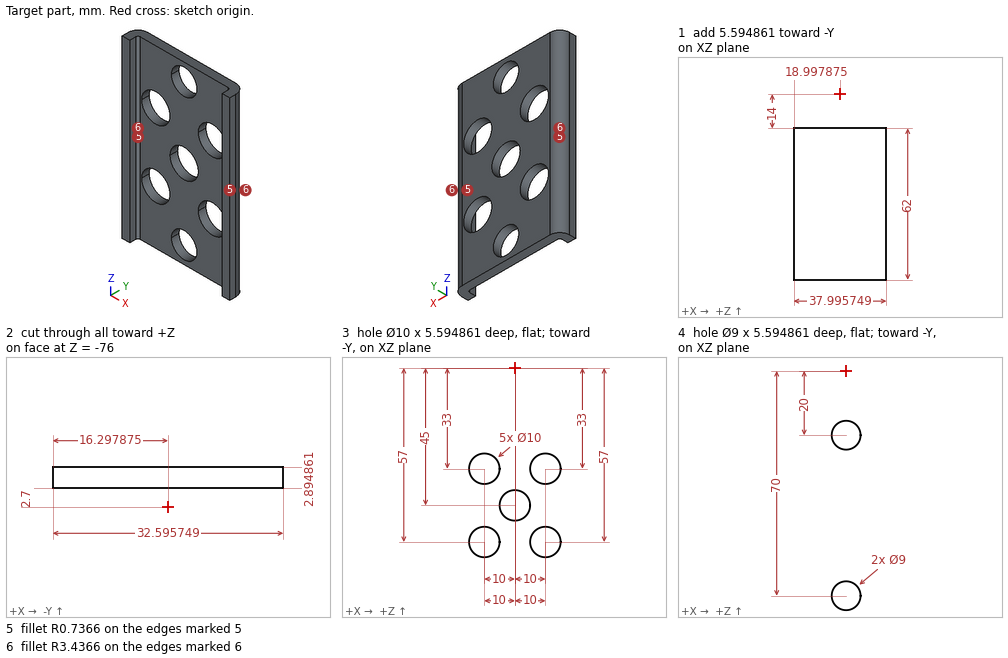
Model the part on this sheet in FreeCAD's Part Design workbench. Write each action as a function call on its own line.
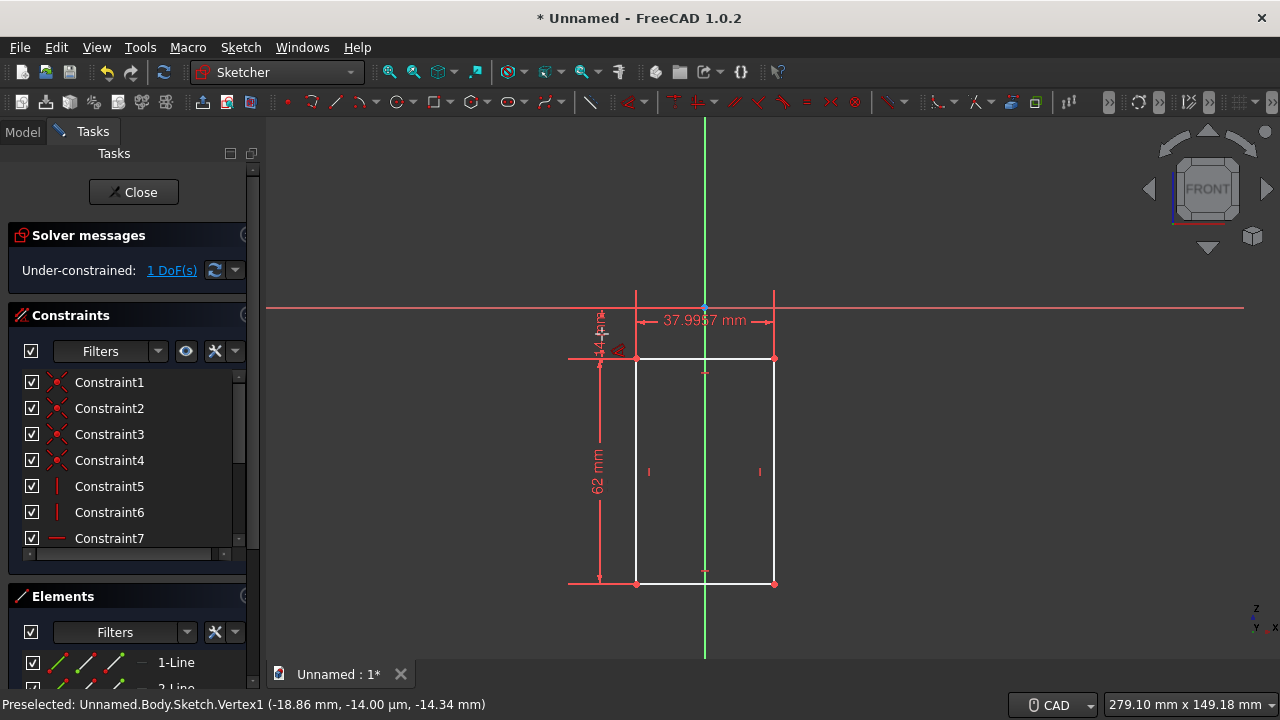
click(636, 359)
click(670, 274)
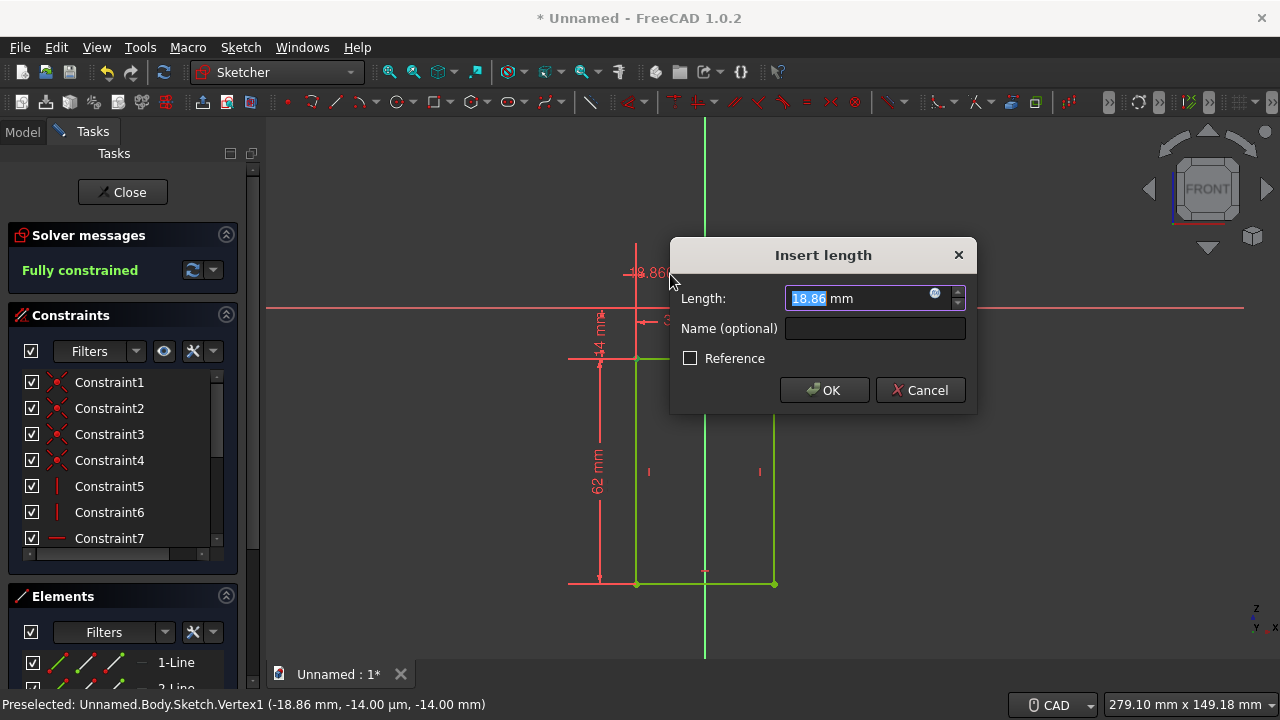
text(18.997875)
key(Return)
key(Escape)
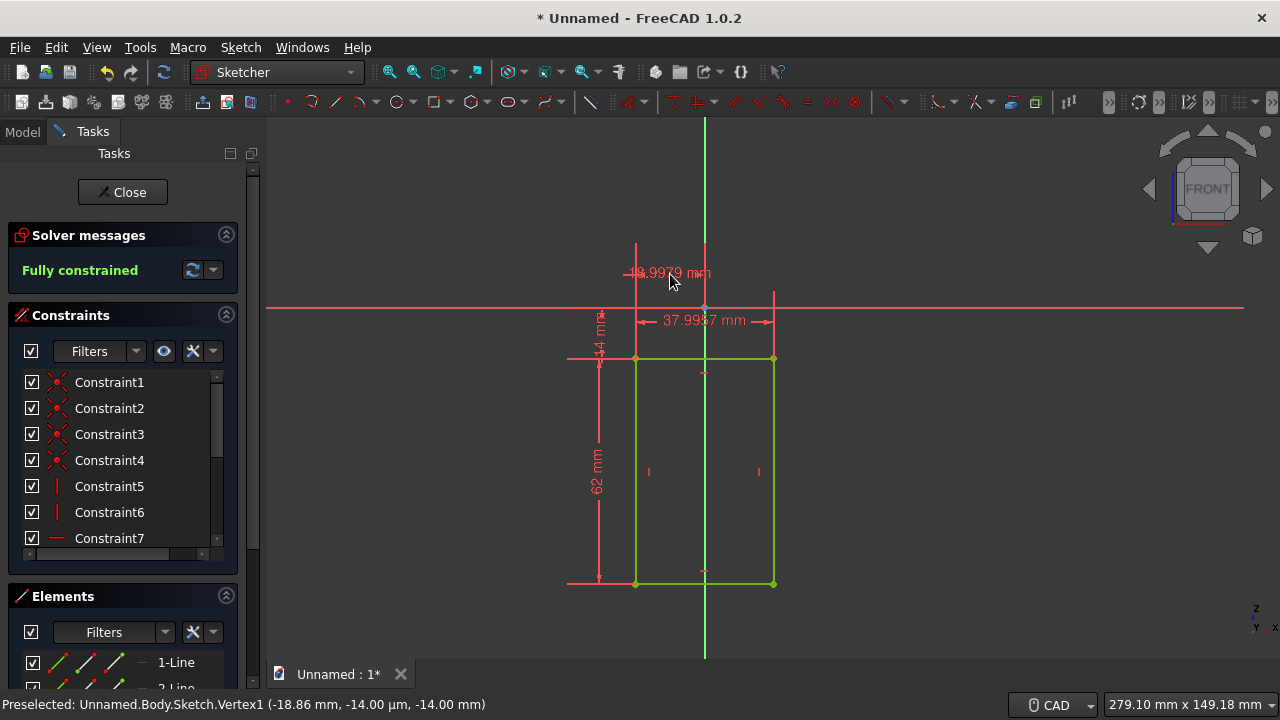
click(123, 192)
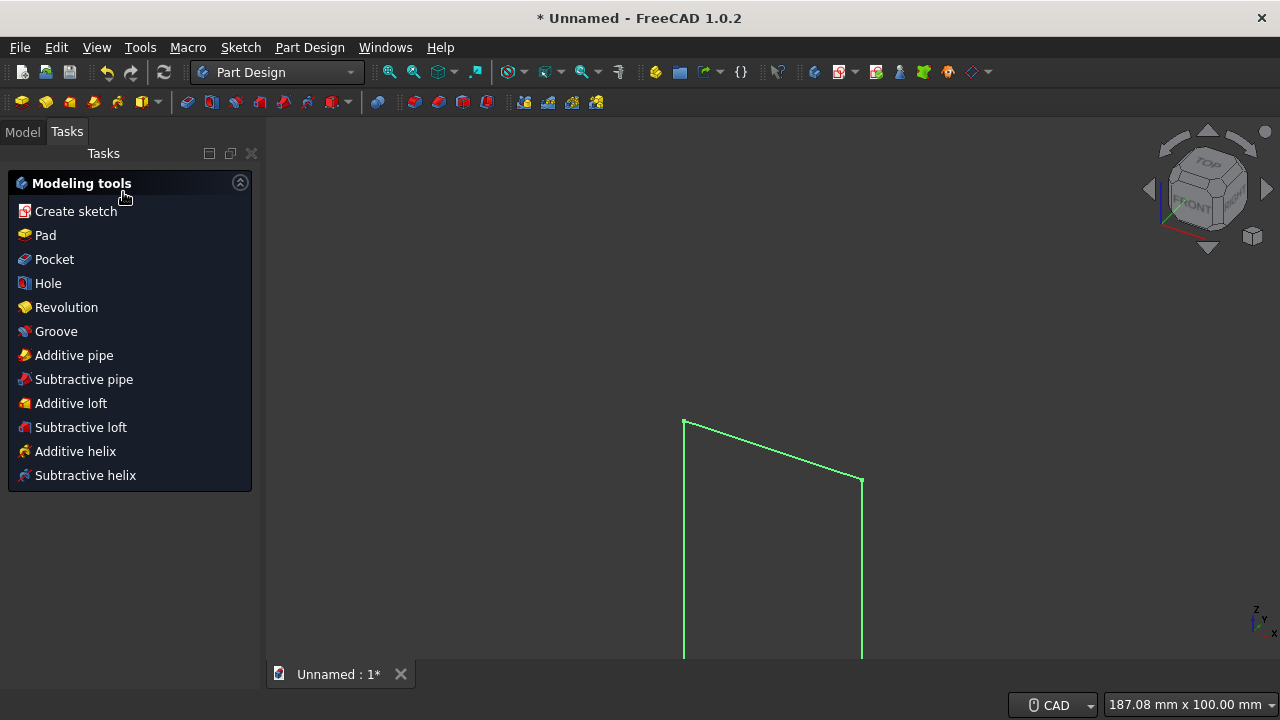
click(22, 102)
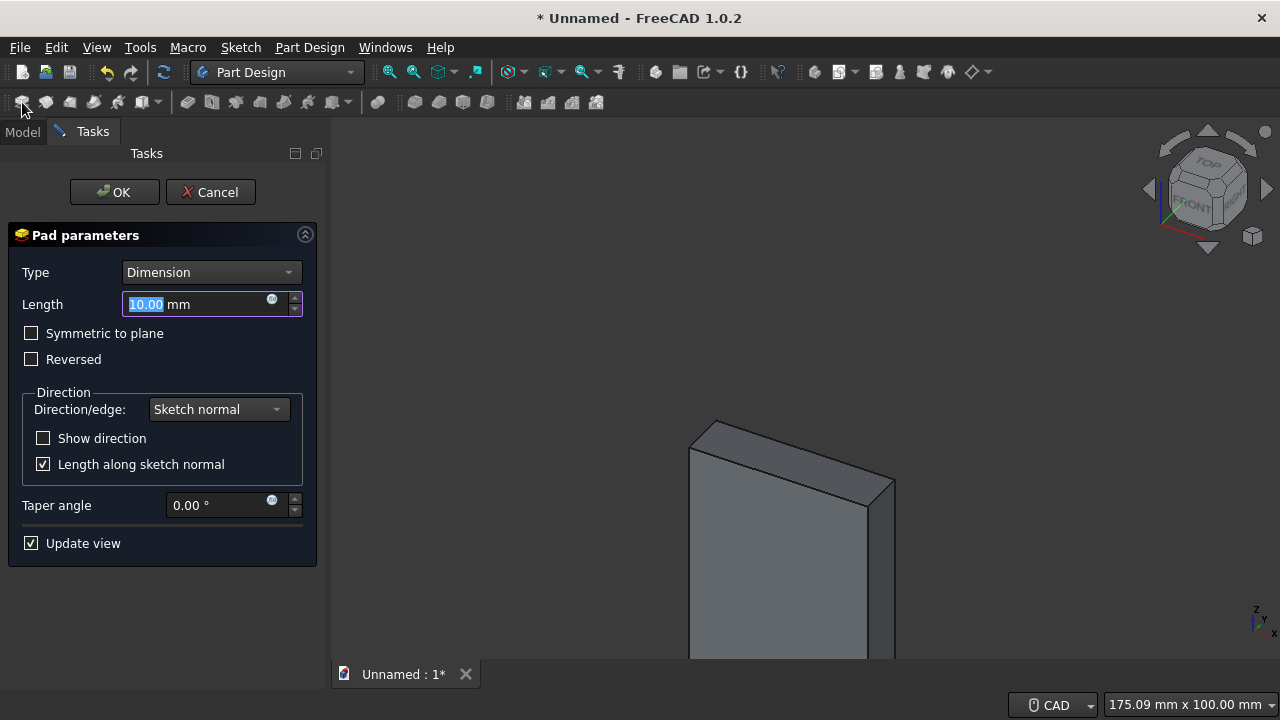
text(5.594861)
key(Tab)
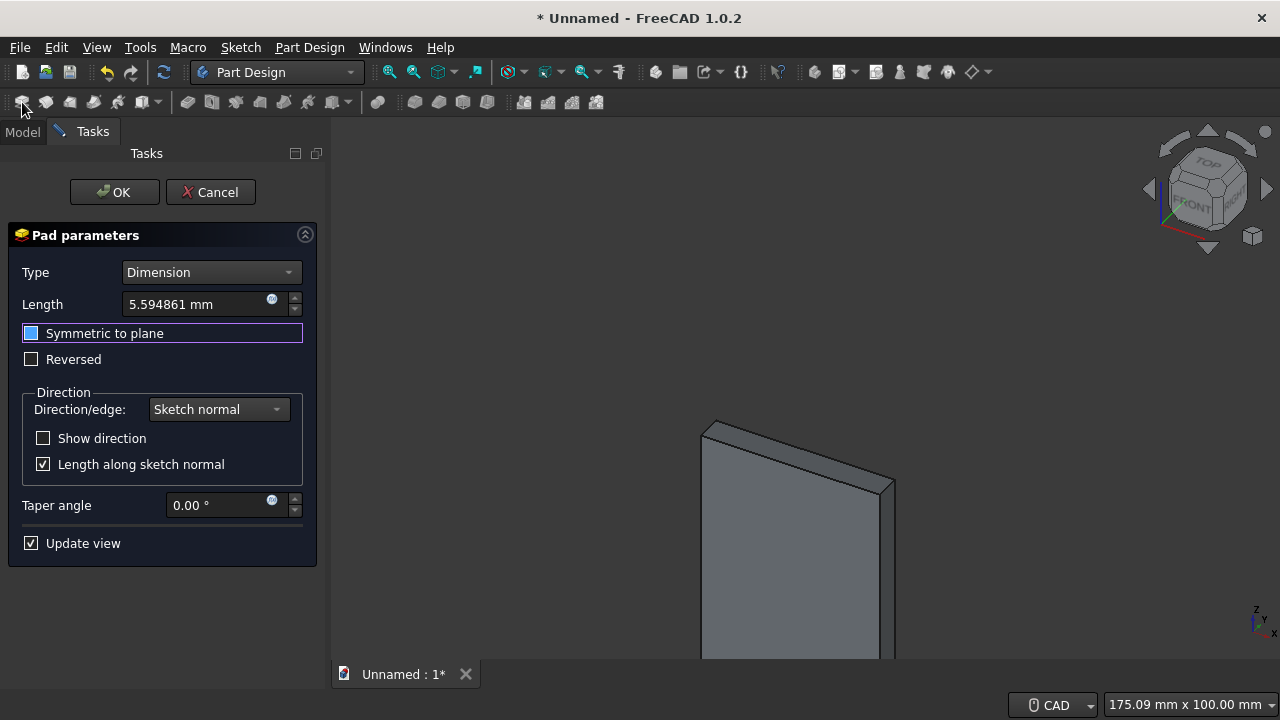
click(115, 192)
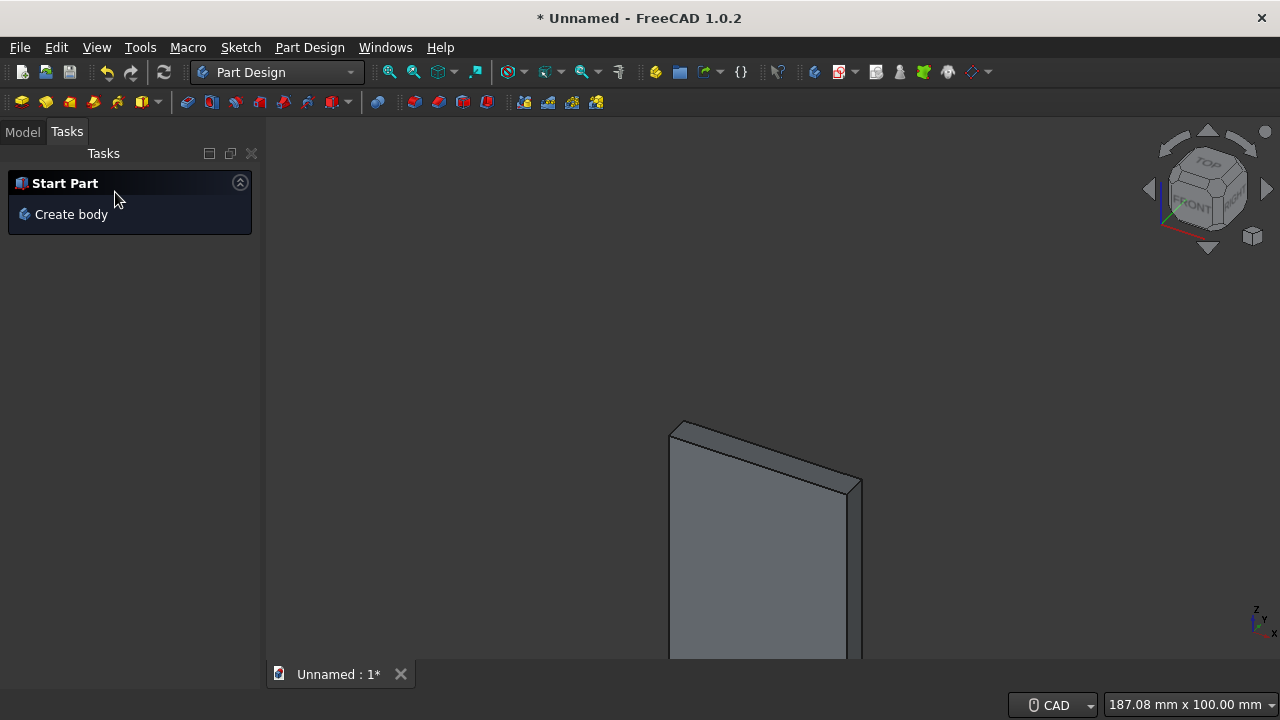
key(v)
key(f)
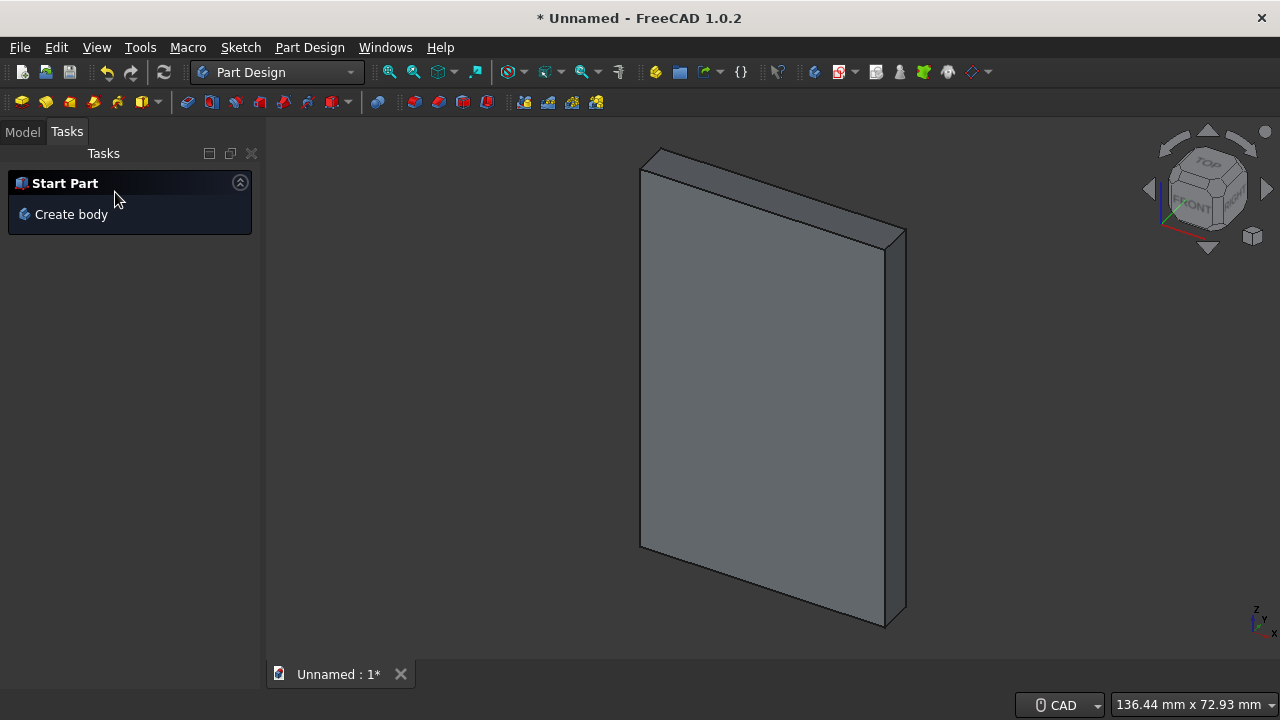
key(5)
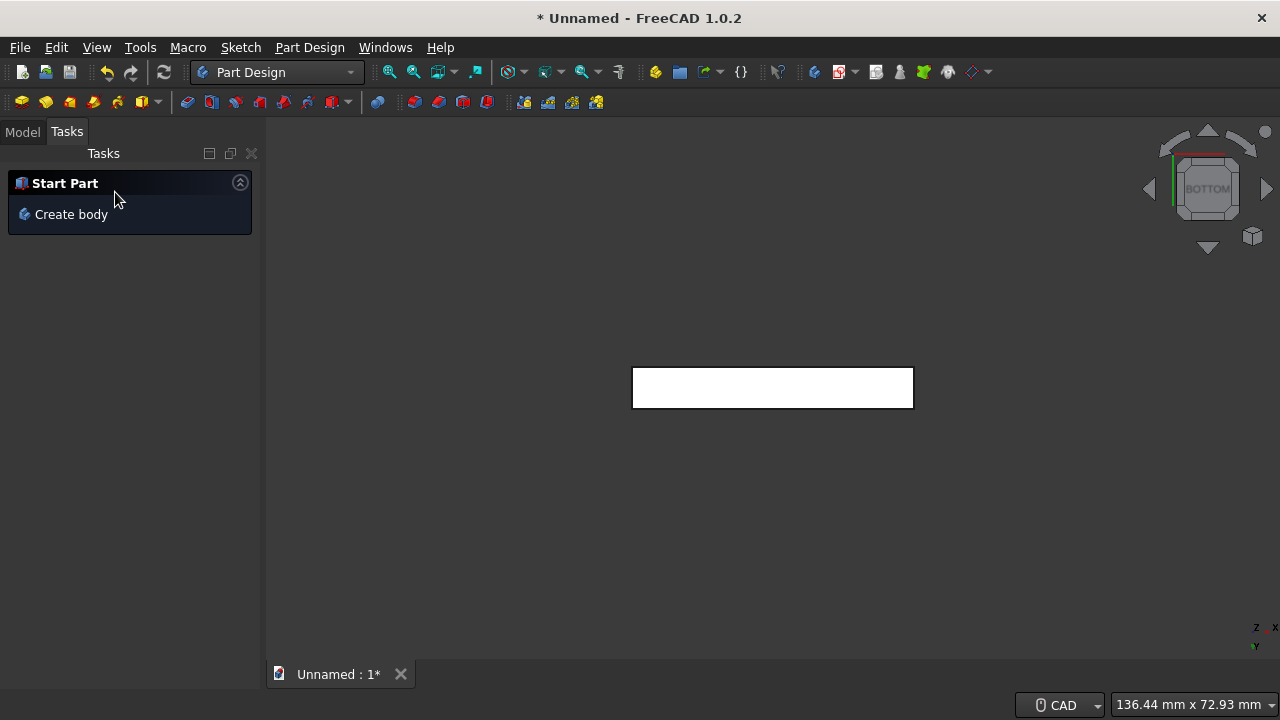
key(v)
key(f)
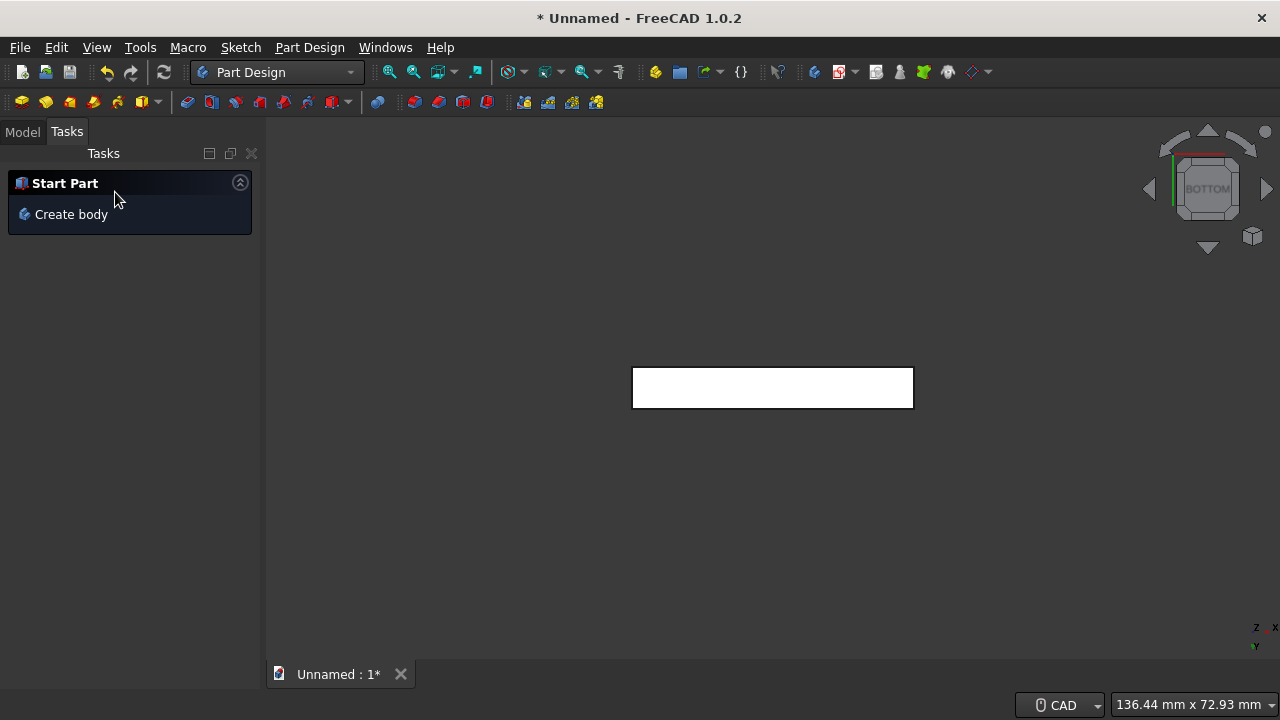
click(854, 387)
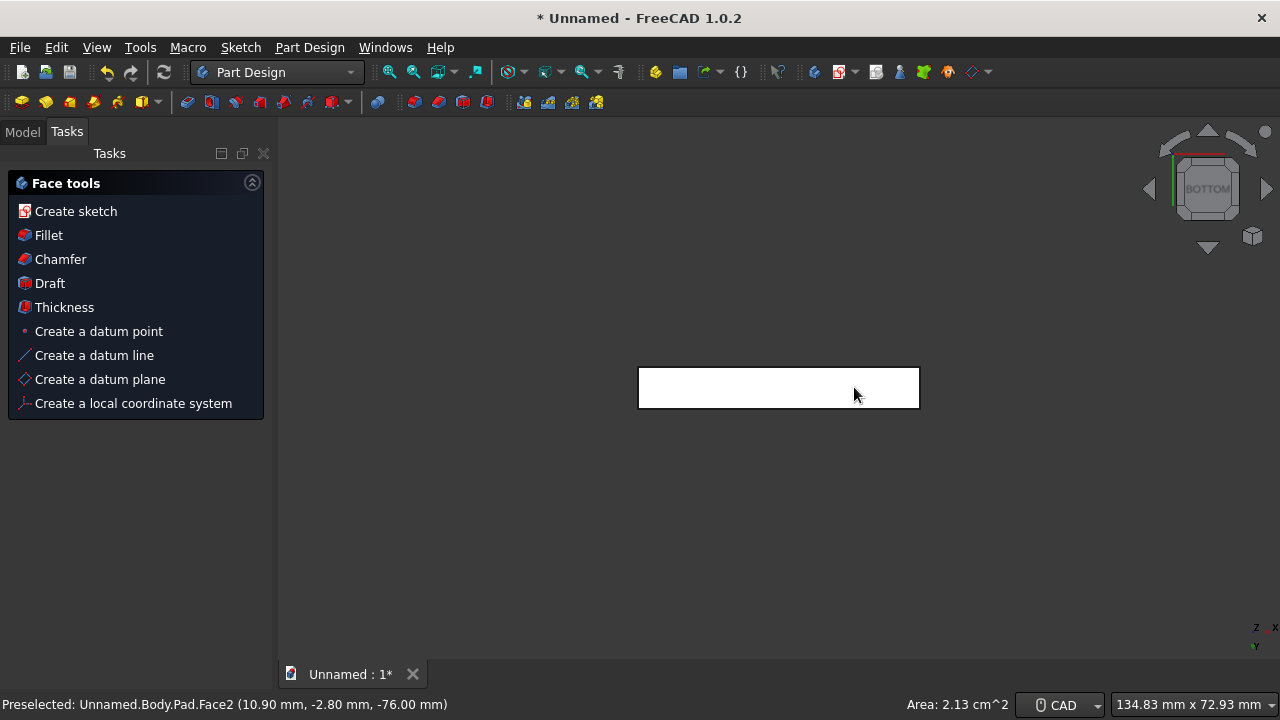
click(840, 72)